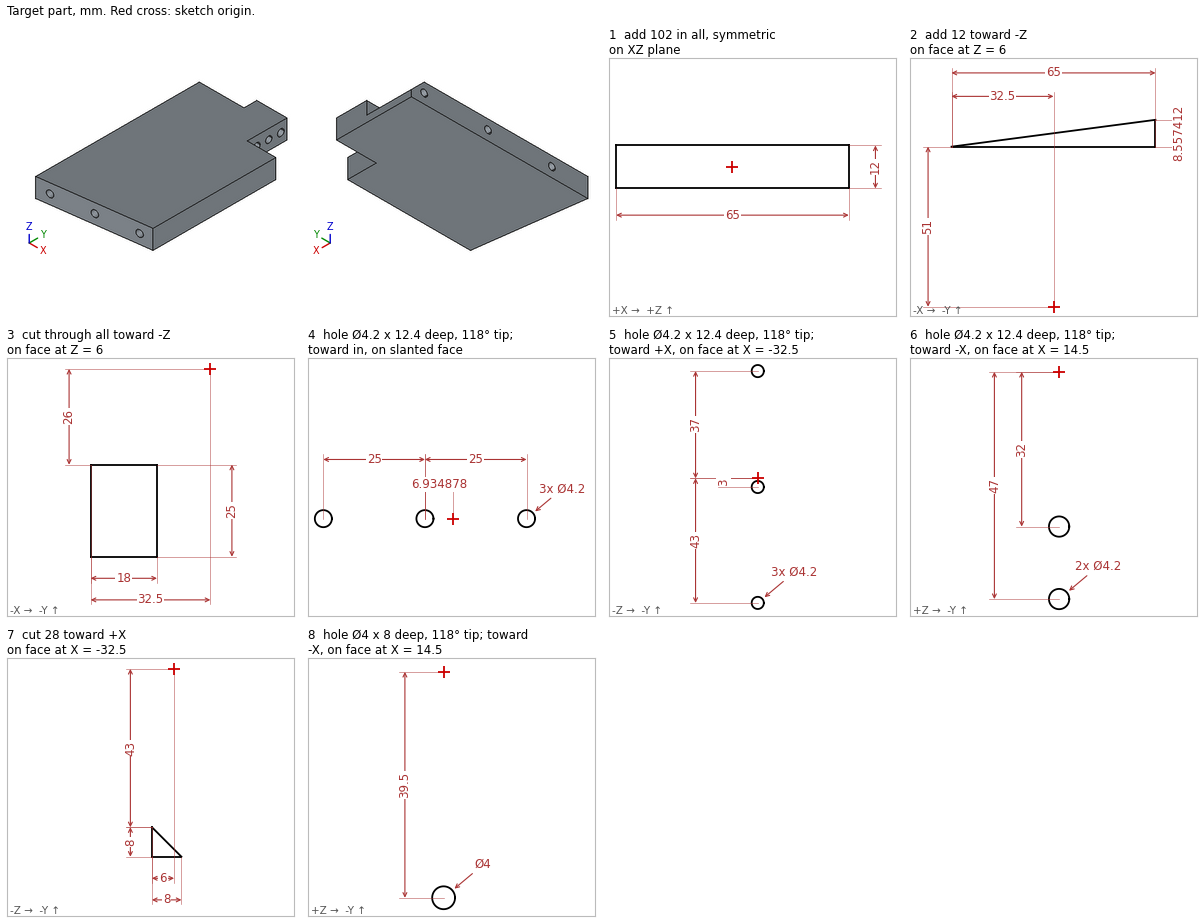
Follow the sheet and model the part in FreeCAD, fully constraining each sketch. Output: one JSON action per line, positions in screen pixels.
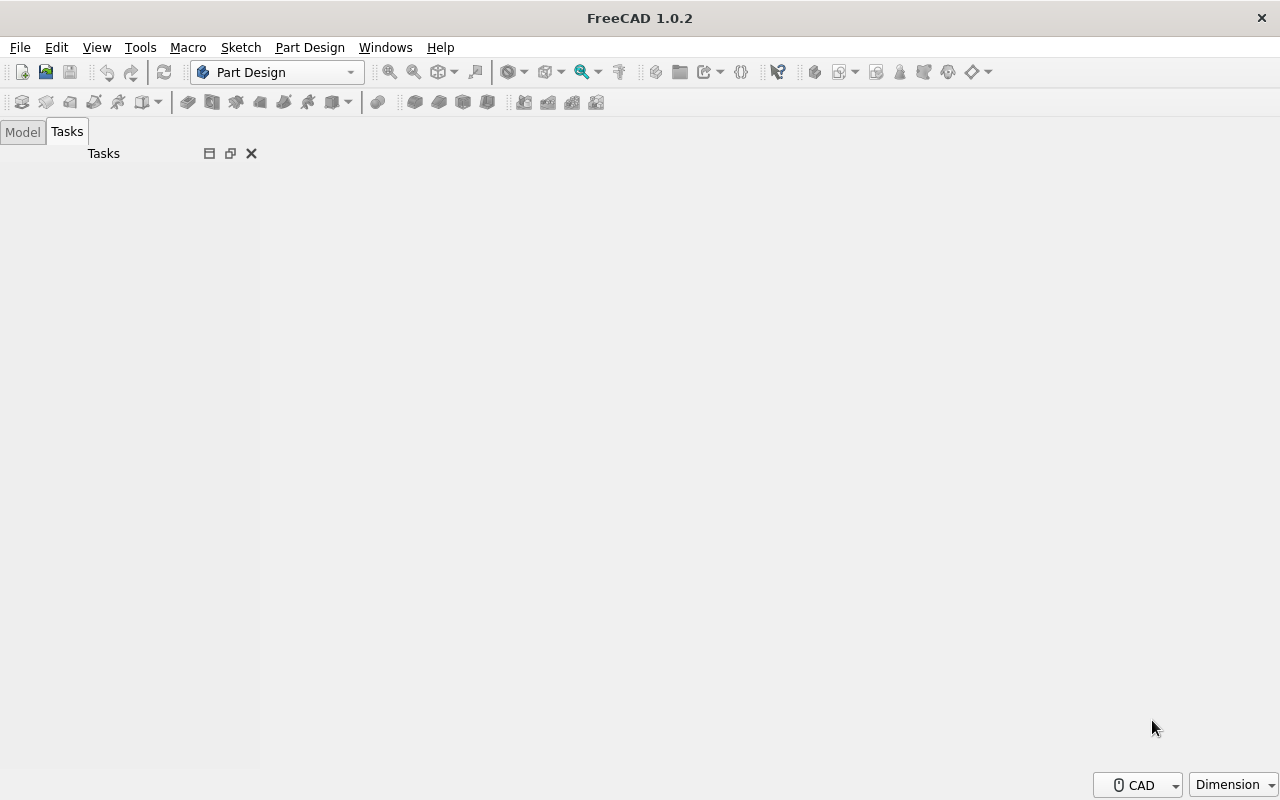
{"action": "left_click", "coordinate": [22, 72]}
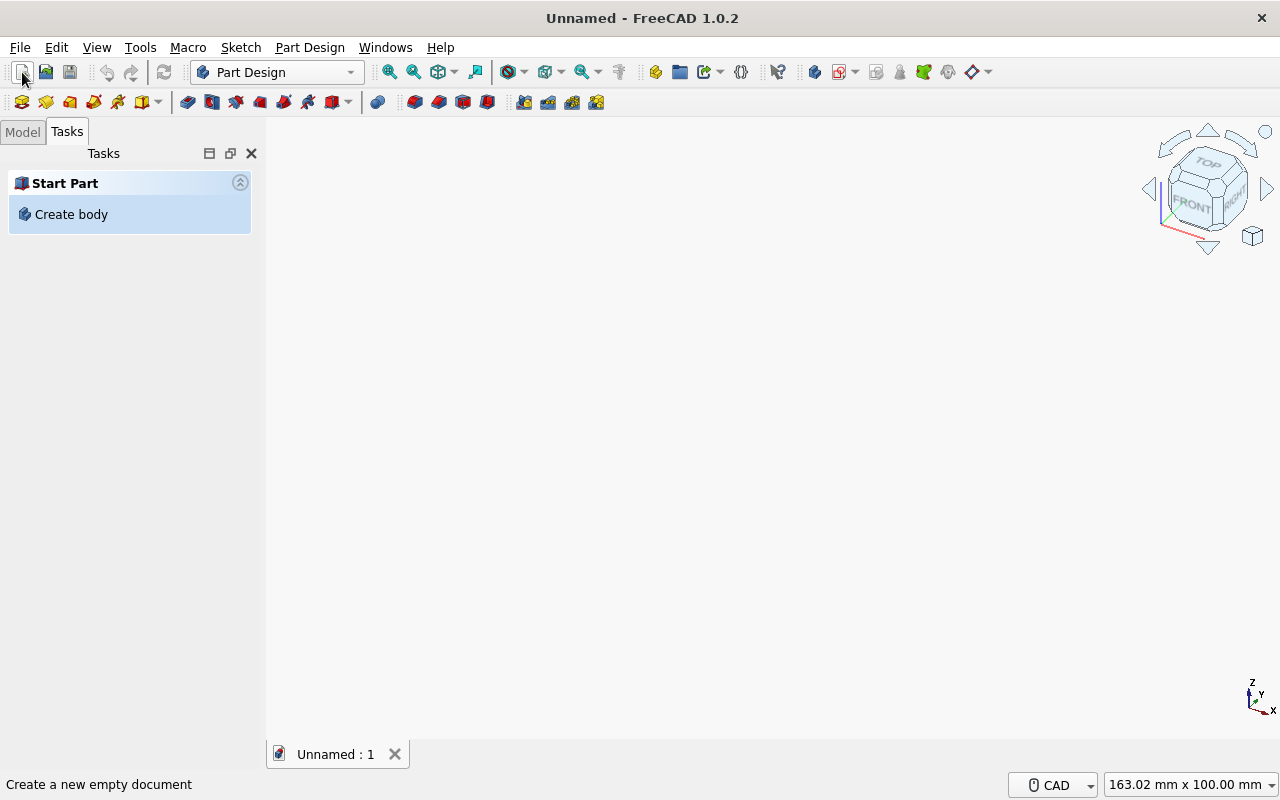
{"action": "left_click", "coordinate": [840, 72]}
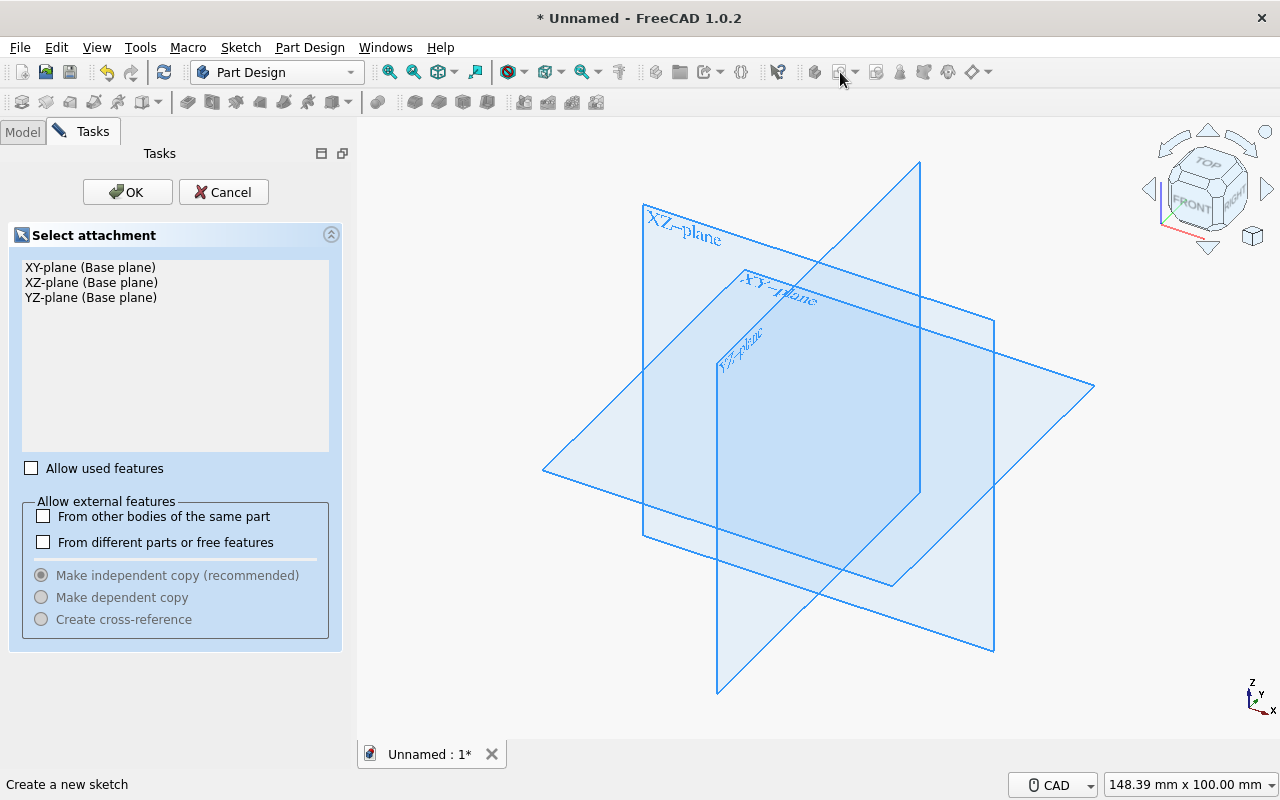
{"action": "left_click", "coordinate": [82, 282]}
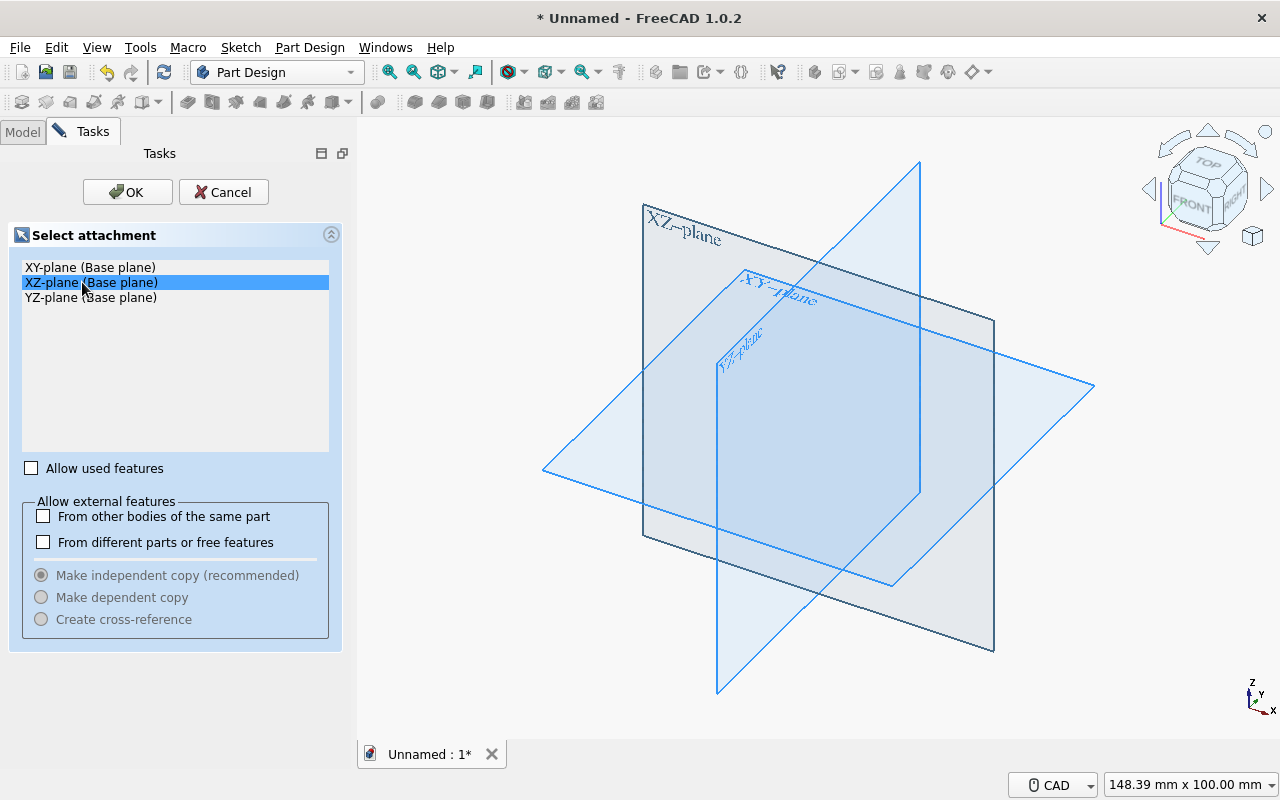
{"action": "left_click", "coordinate": [128, 192]}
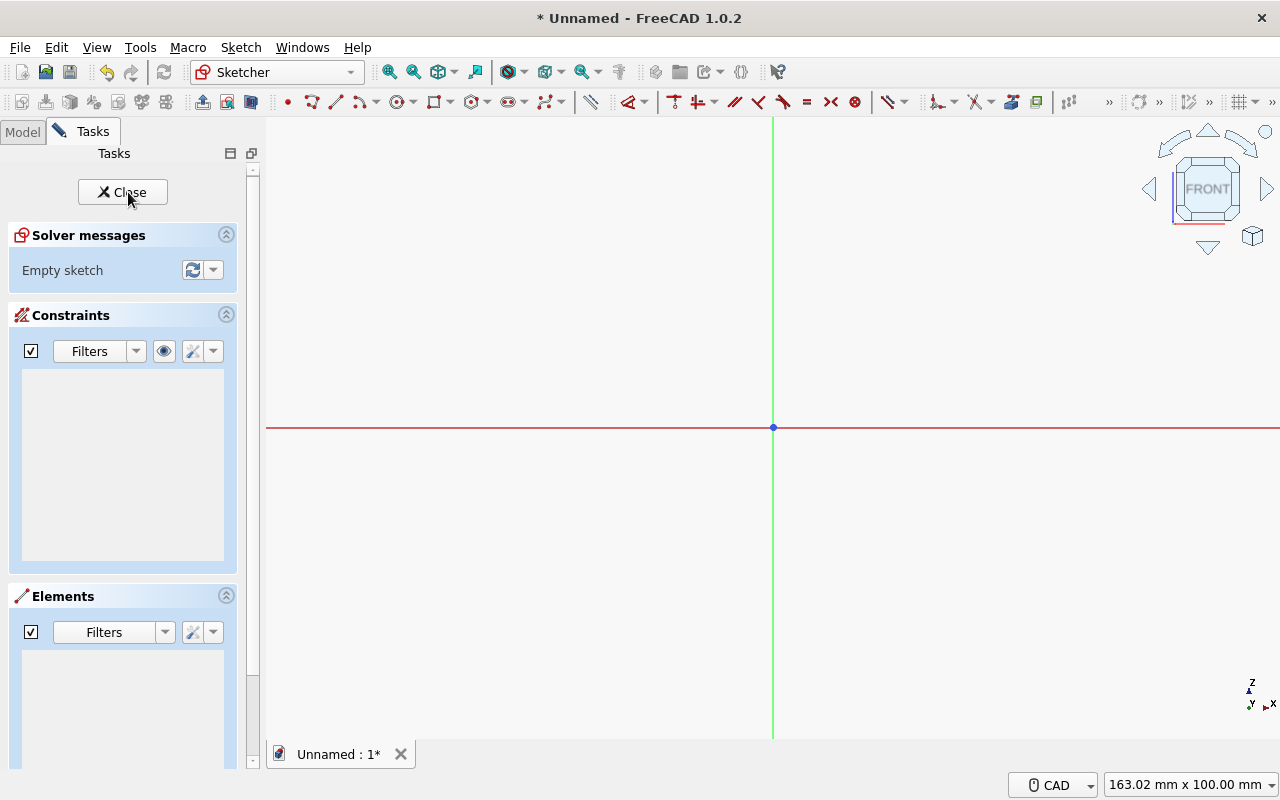
{"action": "scroll", "coordinate": [912, 428], "scroll_direction": "up", "scroll_amount": 2}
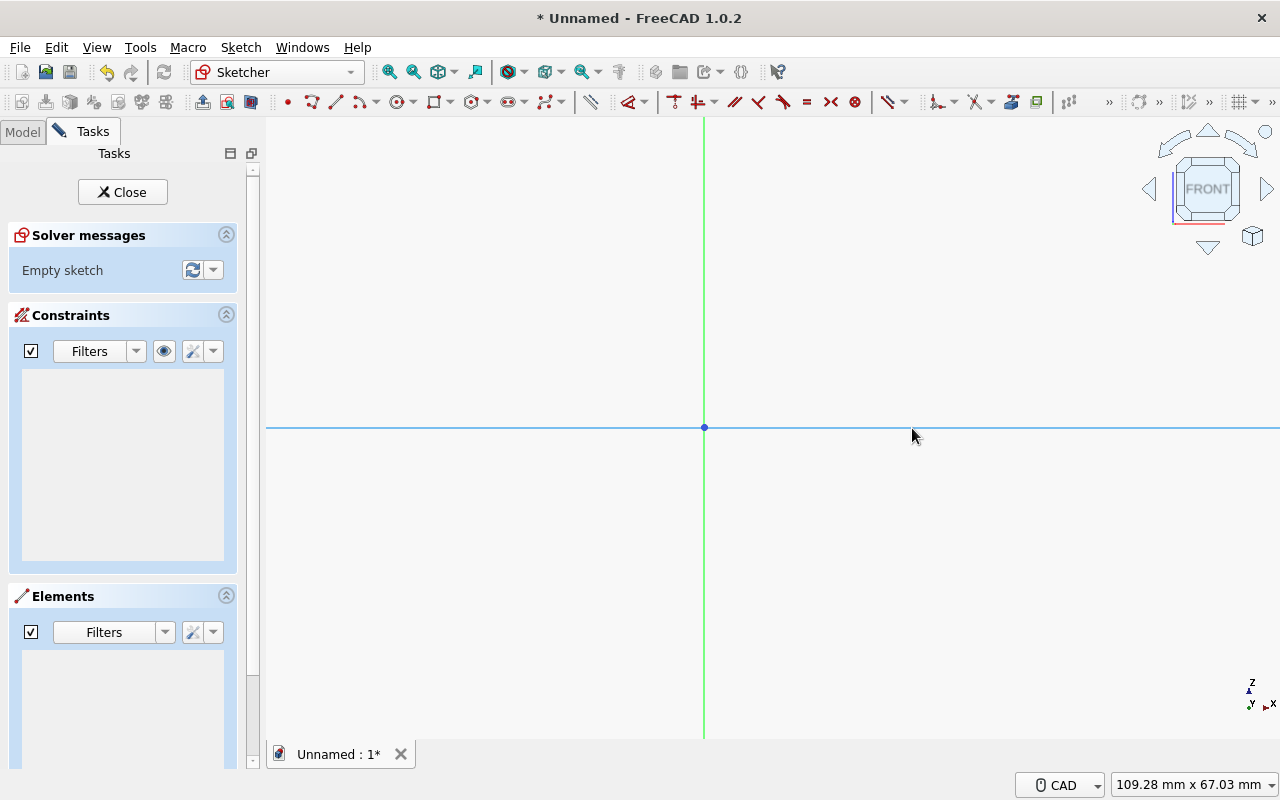
{"action": "key", "text": "g v"}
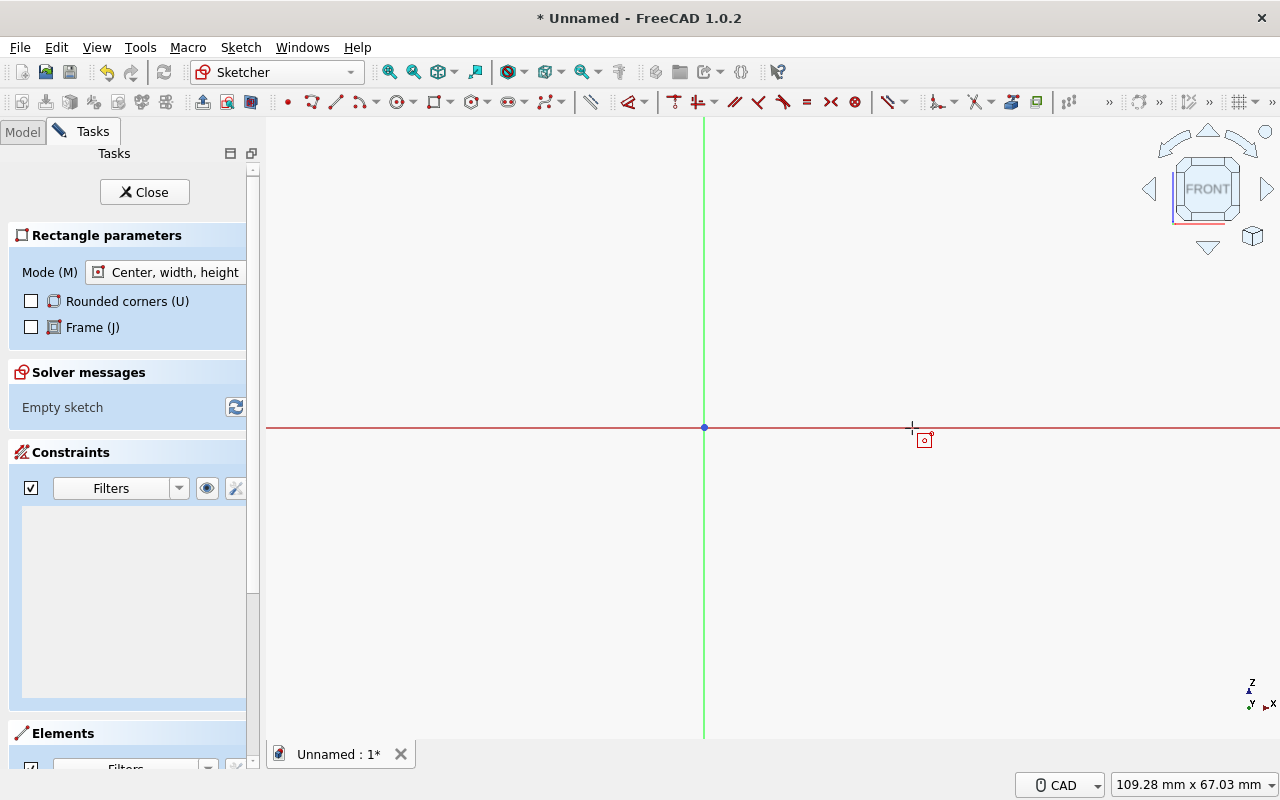
{"action": "left_click", "coordinate": [704, 428]}
{"action": "mouse_move", "coordinate": [1006, 372]}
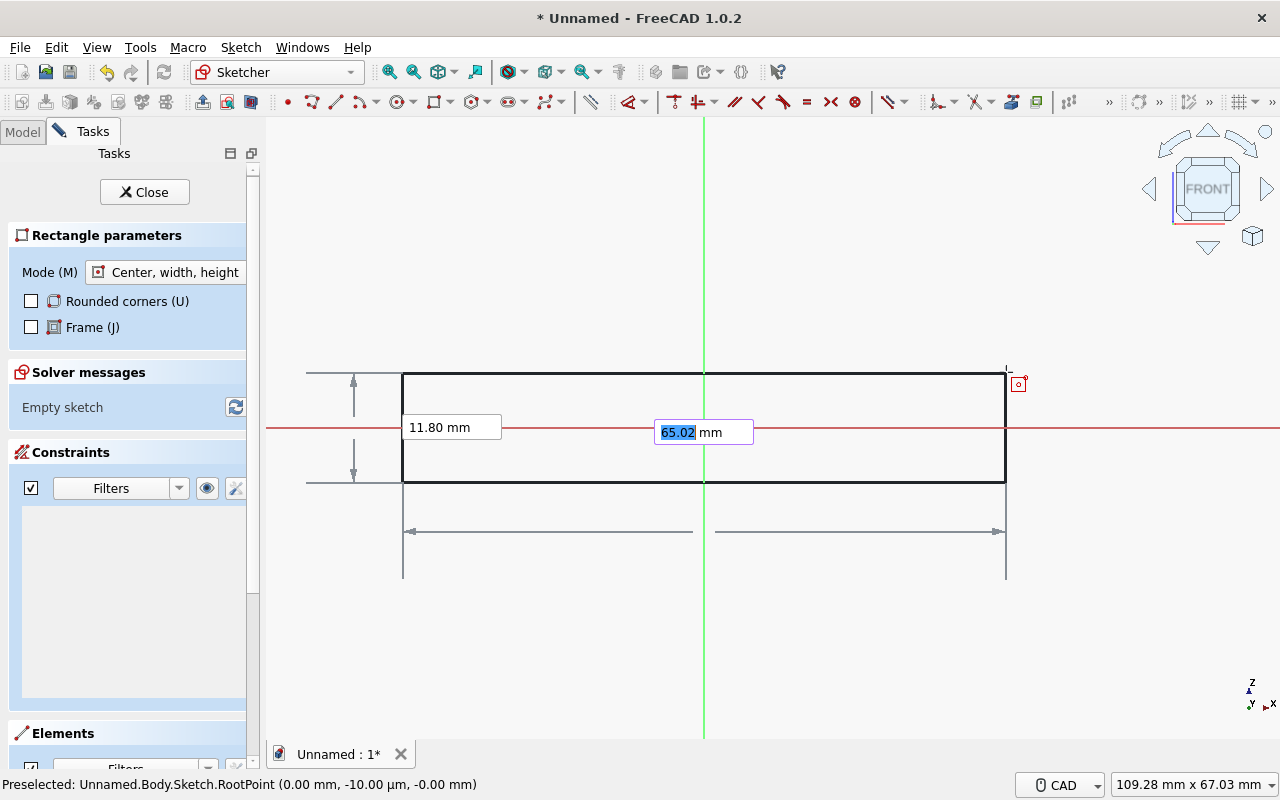
{"action": "type", "text": "65"}
{"action": "key", "text": "Tab"}
{"action": "type", "text": "12"}
{"action": "key", "text": "Return"}
{"action": "key", "text": "Escape"}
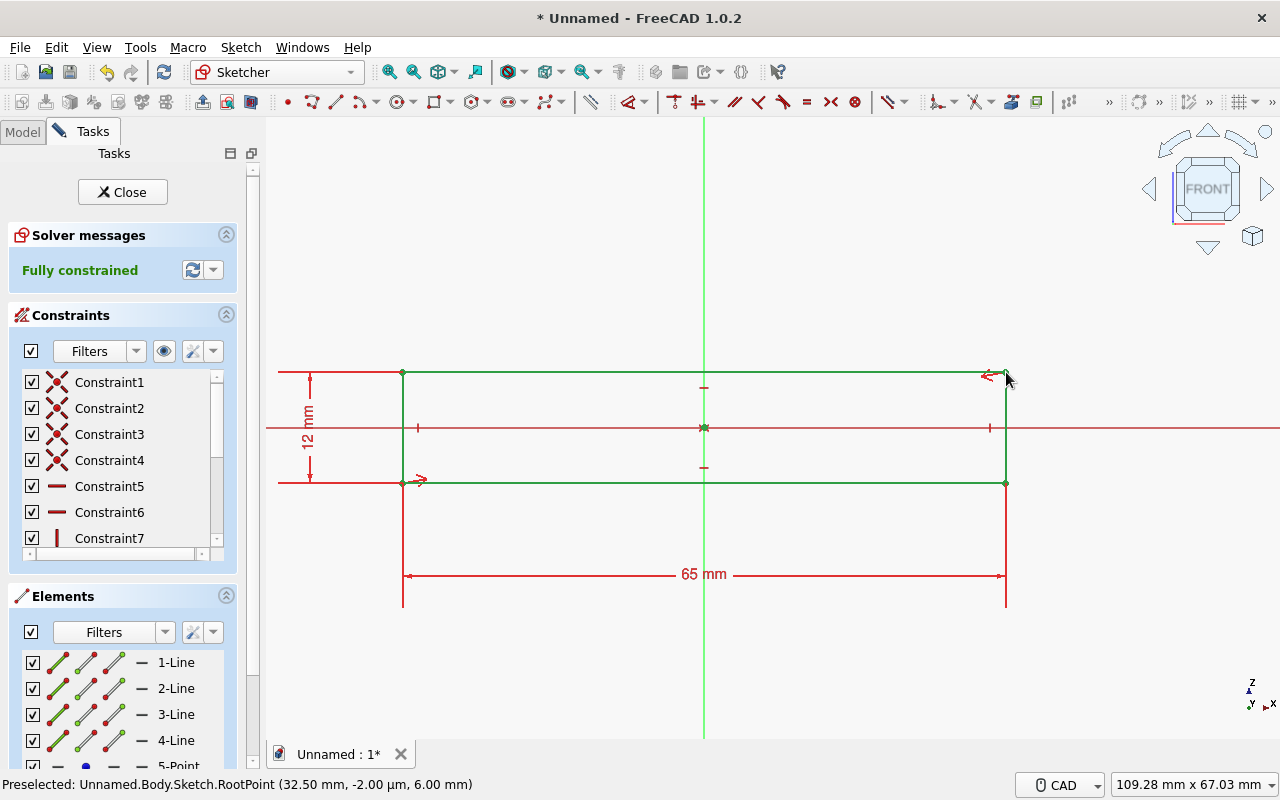
{"action": "left_click", "coordinate": [123, 192]}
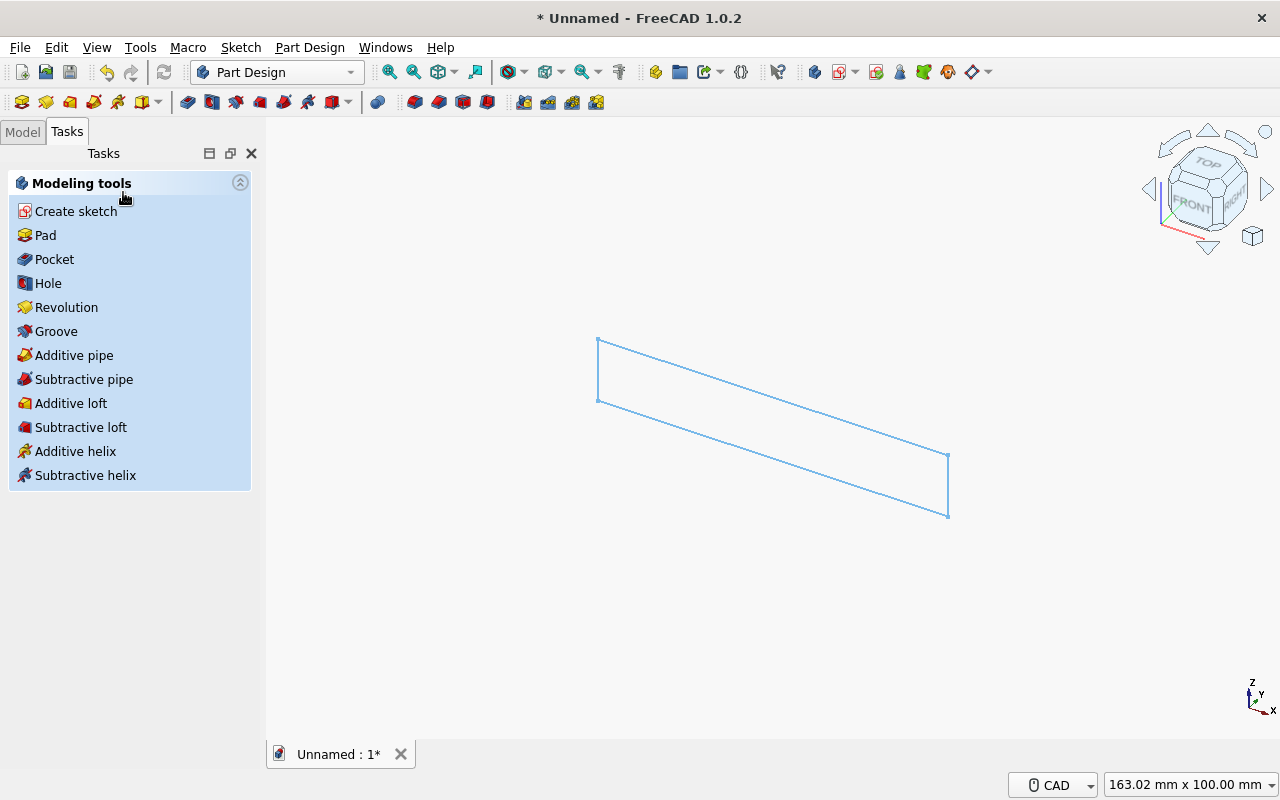
{"action": "left_click", "coordinate": [22, 102]}